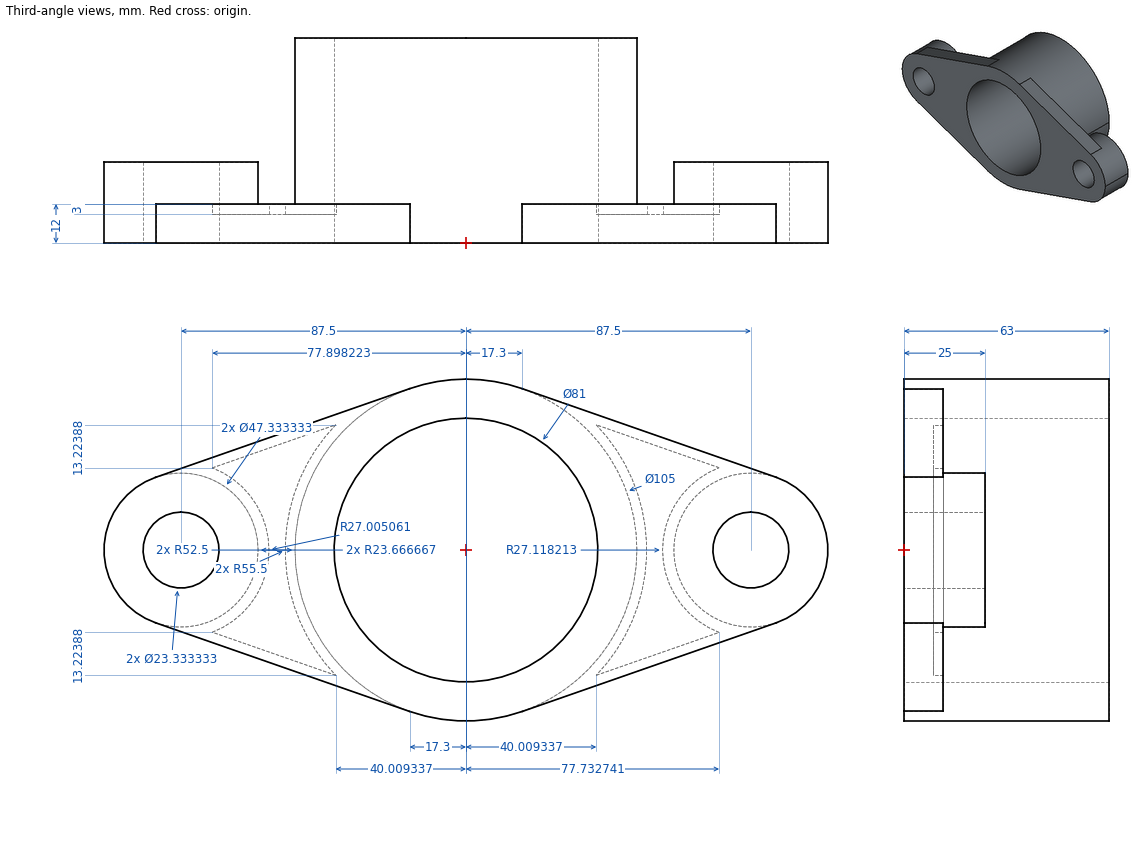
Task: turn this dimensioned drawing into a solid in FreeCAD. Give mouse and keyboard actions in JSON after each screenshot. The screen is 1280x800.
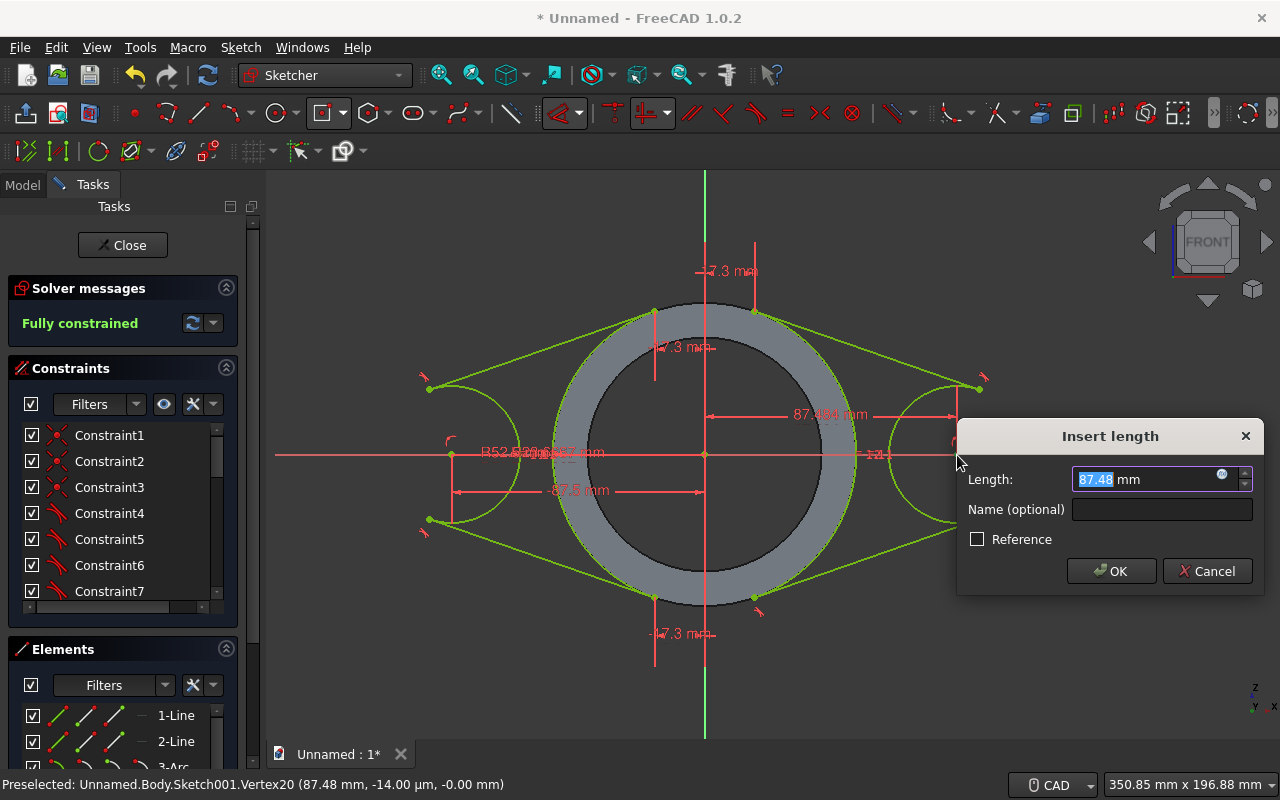
{"action": "type", "text": "87.5"}
{"action": "key", "text": "Return"}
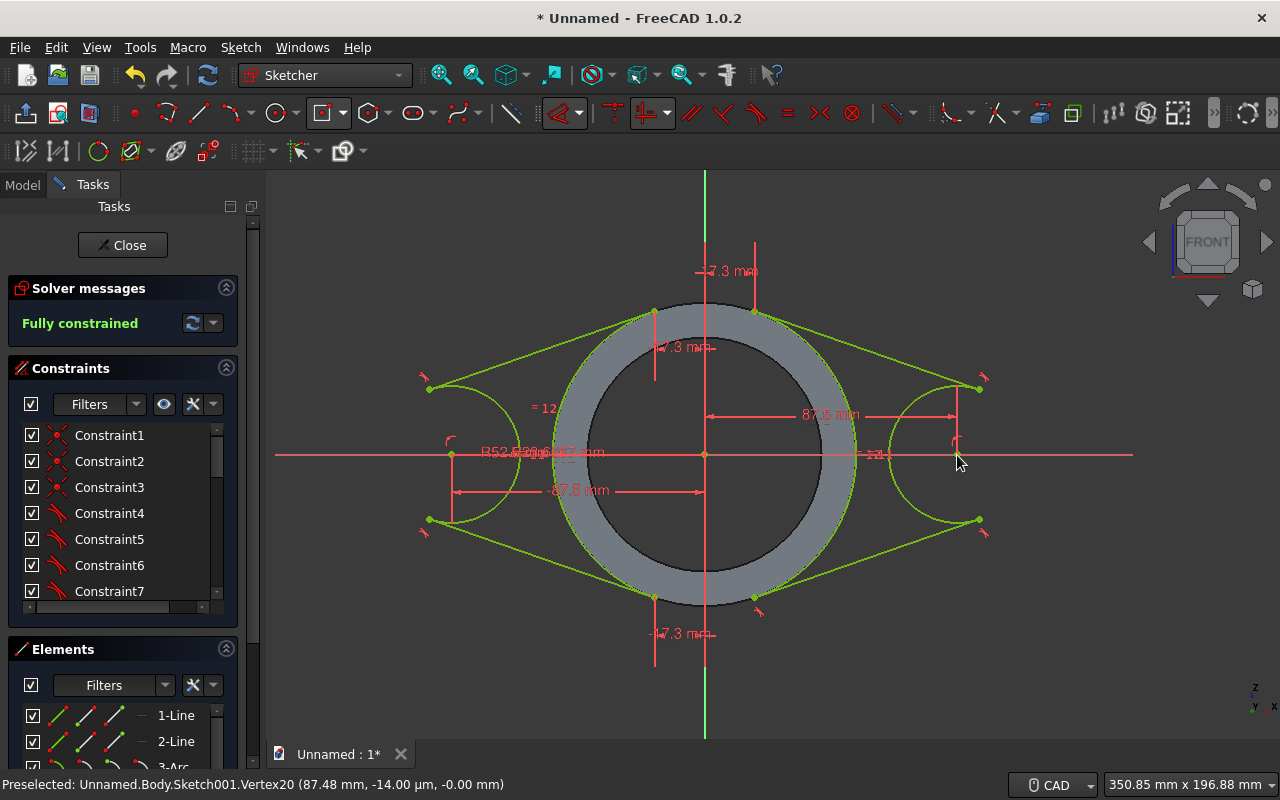
{"action": "left_click", "coordinate": [123, 245]}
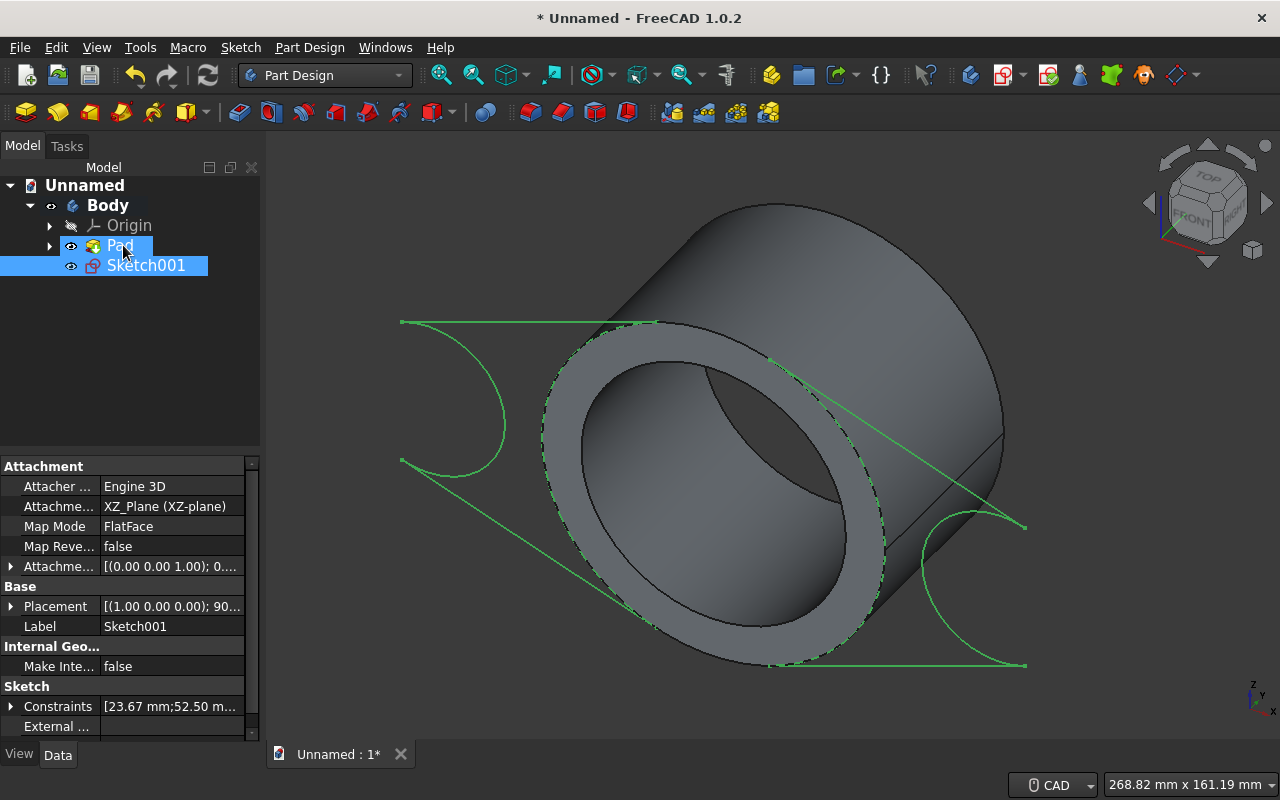
{"action": "left_click", "coordinate": [26, 112]}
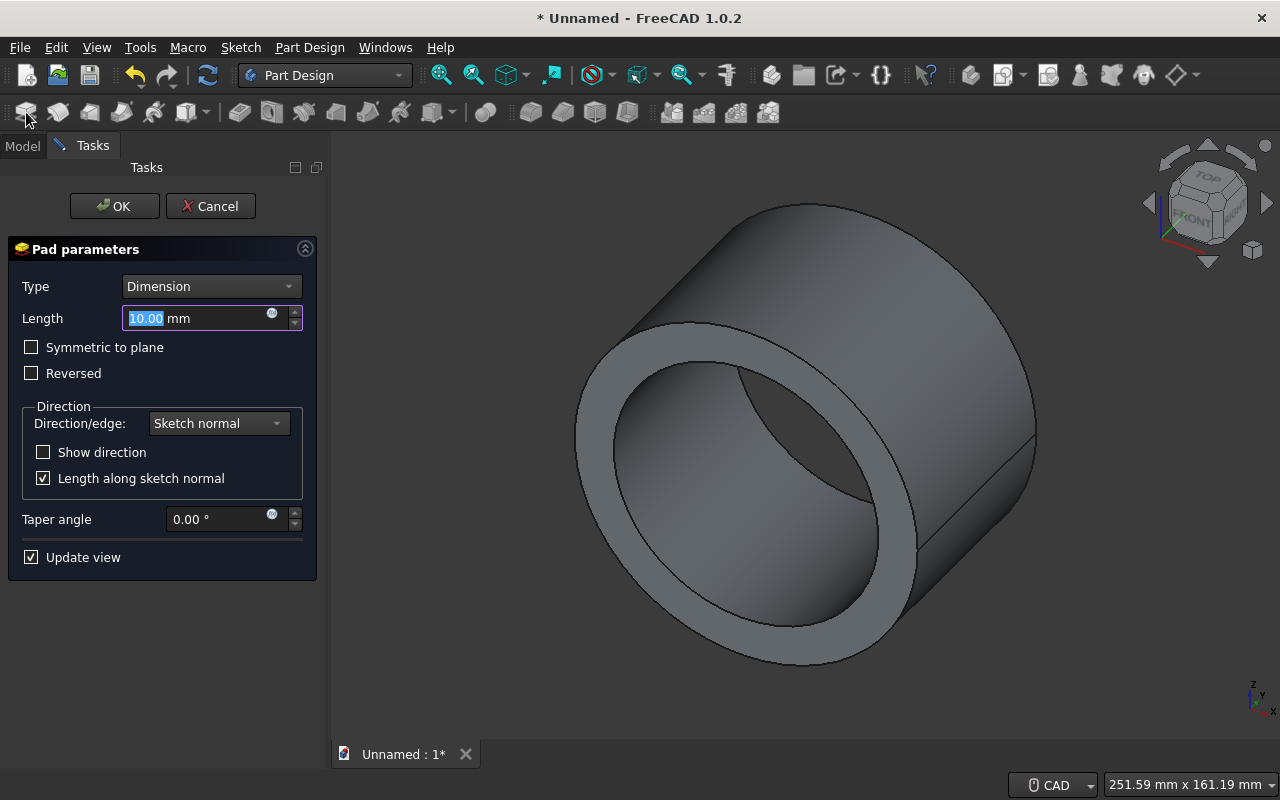
{"action": "type", "text": "12"}
{"action": "key", "text": "Tab"}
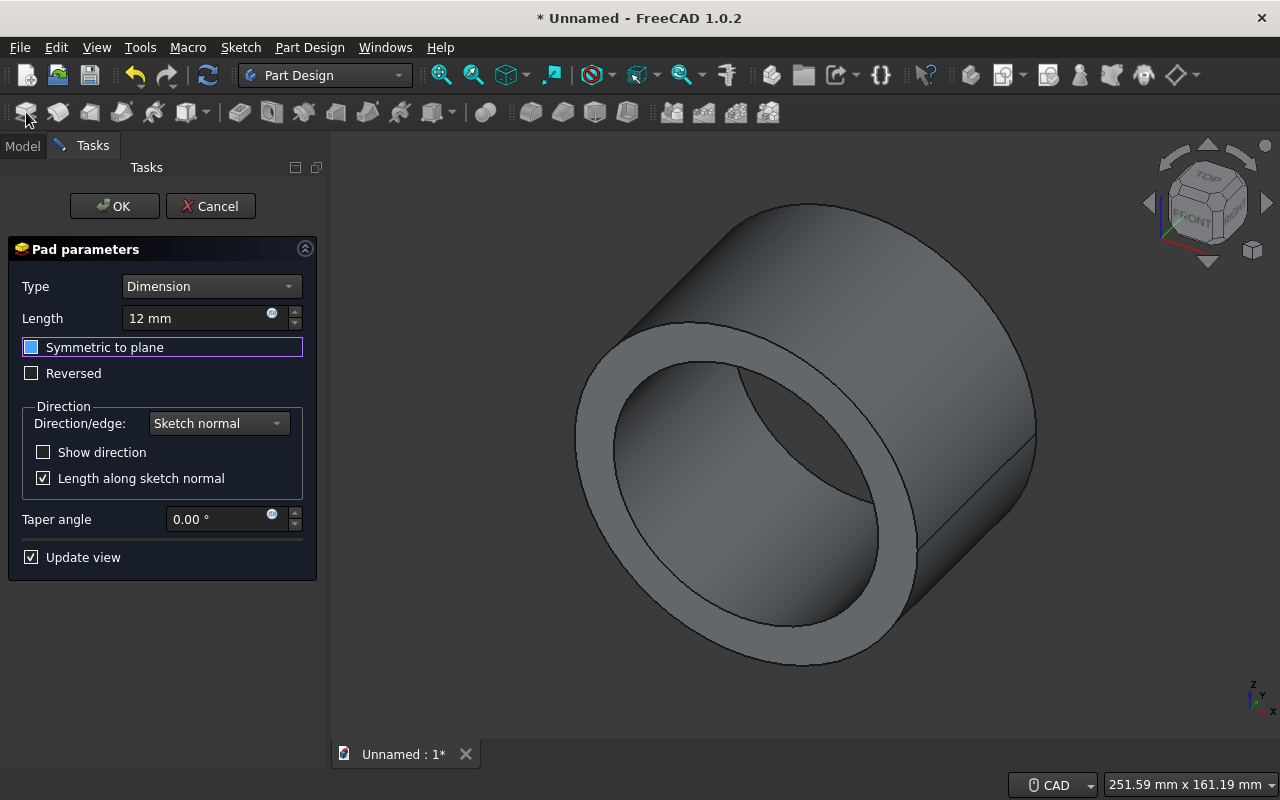
{"action": "left_click", "coordinate": [30, 373]}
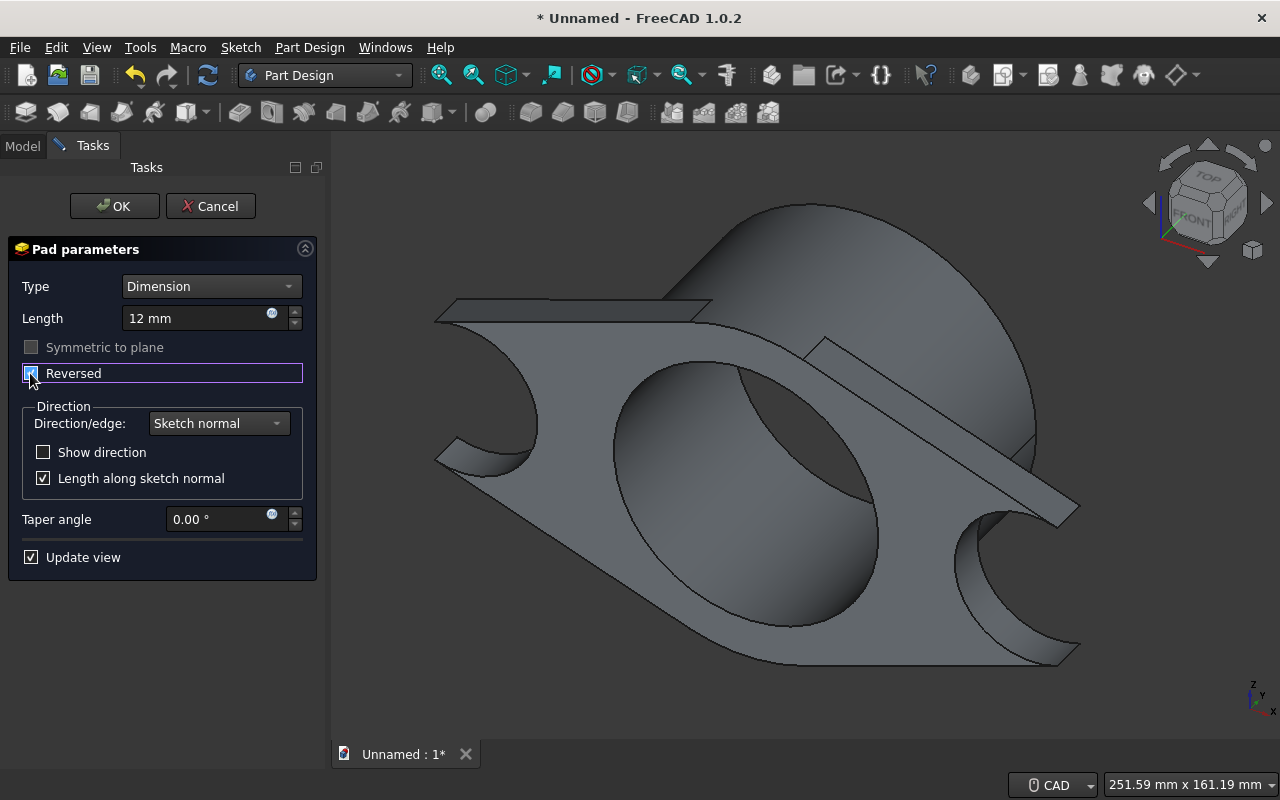
{"action": "left_click", "coordinate": [115, 206]}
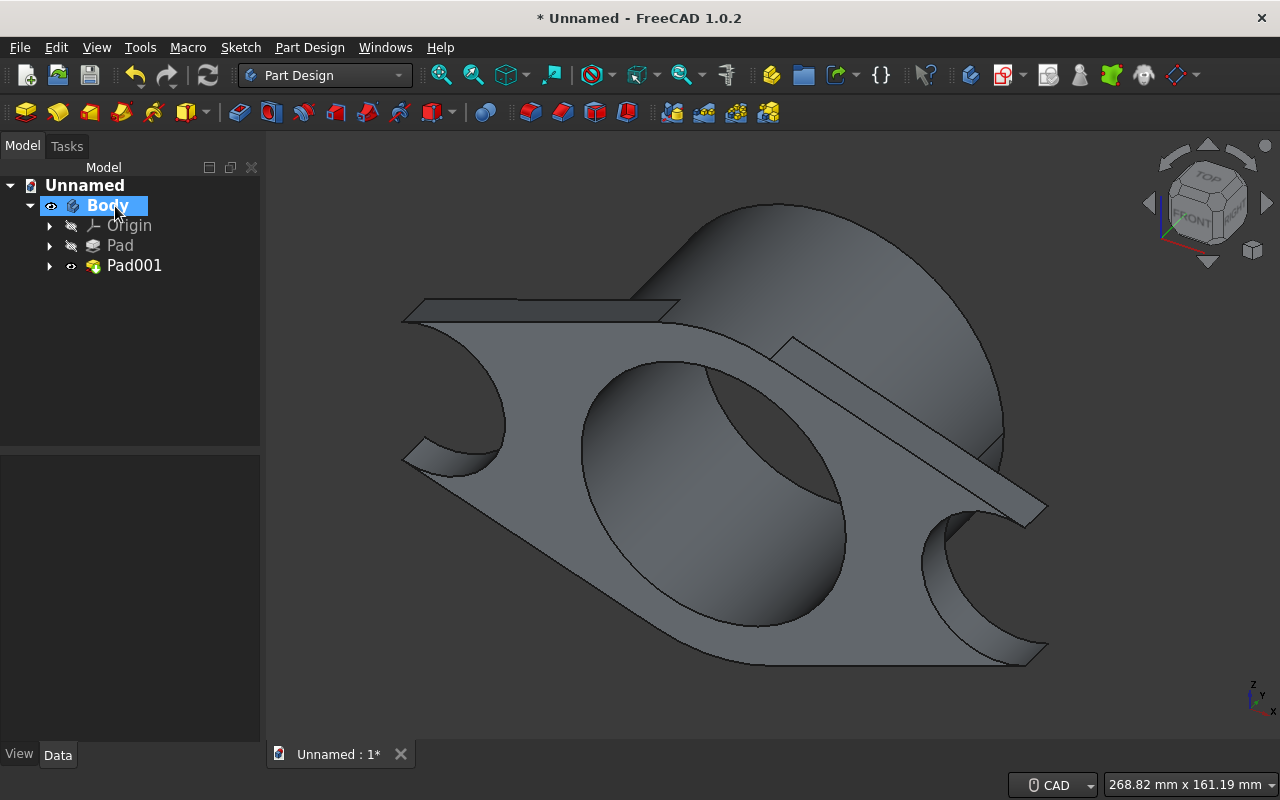
{"action": "key", "text": "v f"}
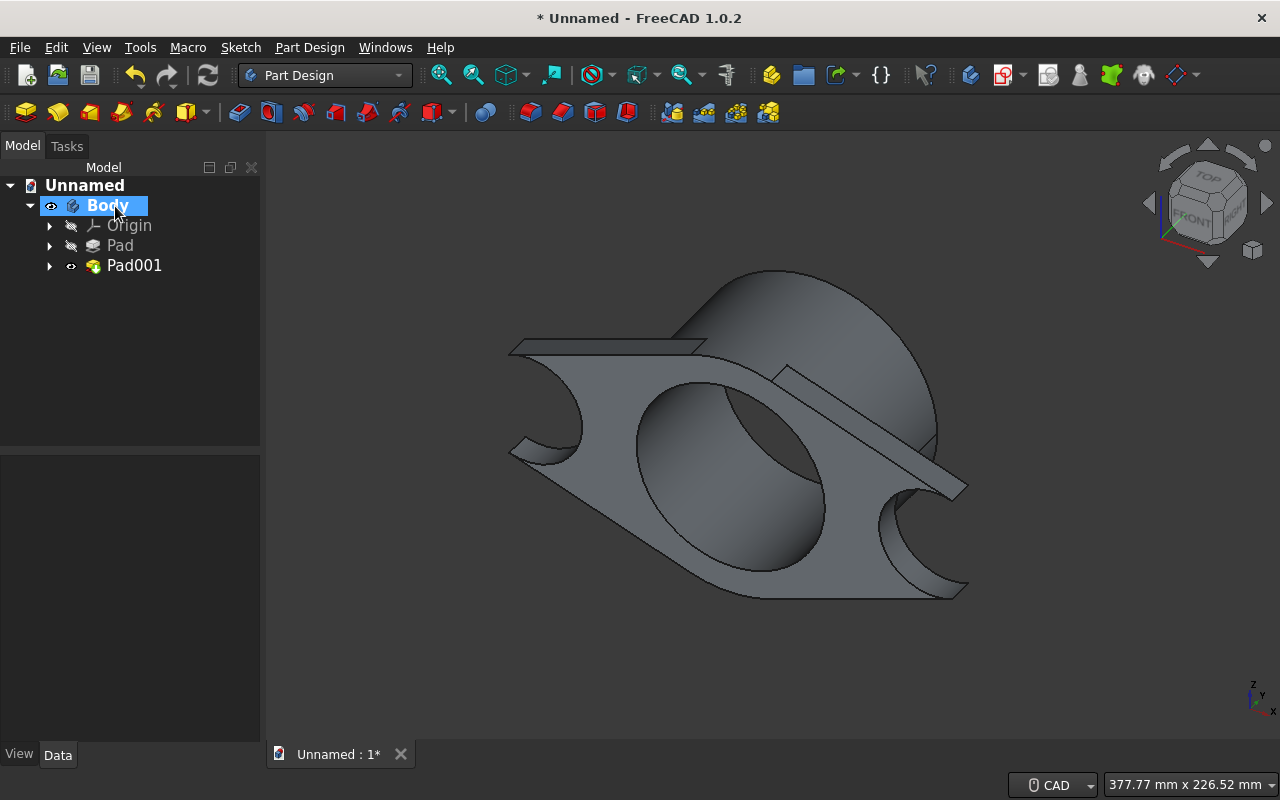
{"action": "left_click", "coordinate": [1004, 76]}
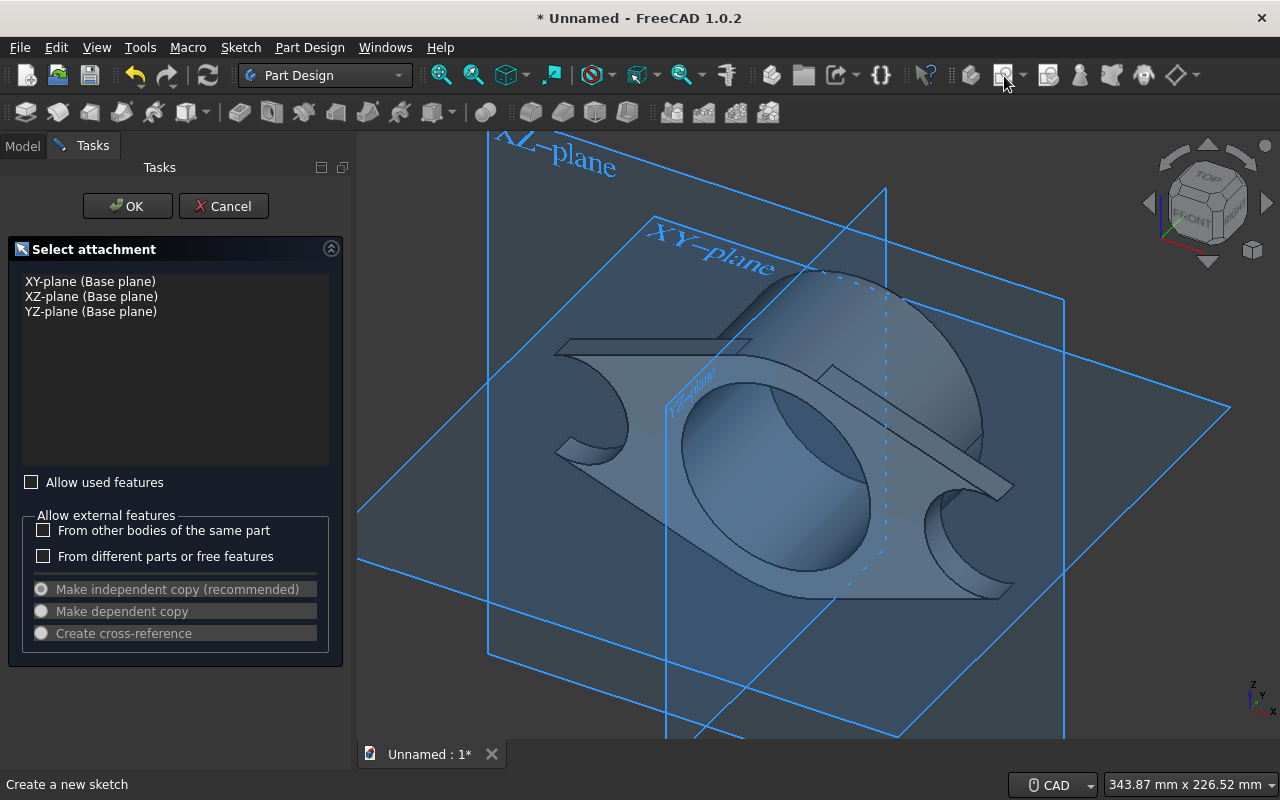
{"action": "left_click", "coordinate": [82, 296]}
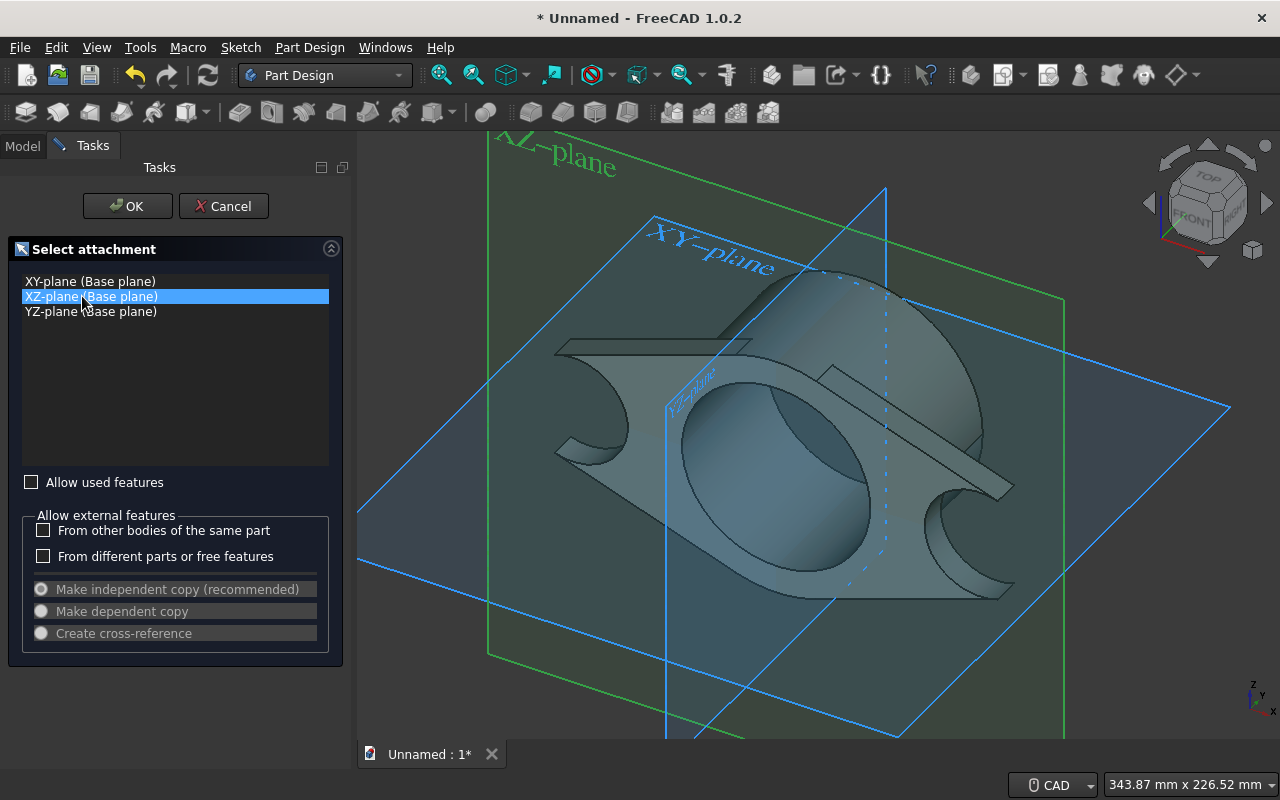
{"action": "left_click", "coordinate": [128, 206]}